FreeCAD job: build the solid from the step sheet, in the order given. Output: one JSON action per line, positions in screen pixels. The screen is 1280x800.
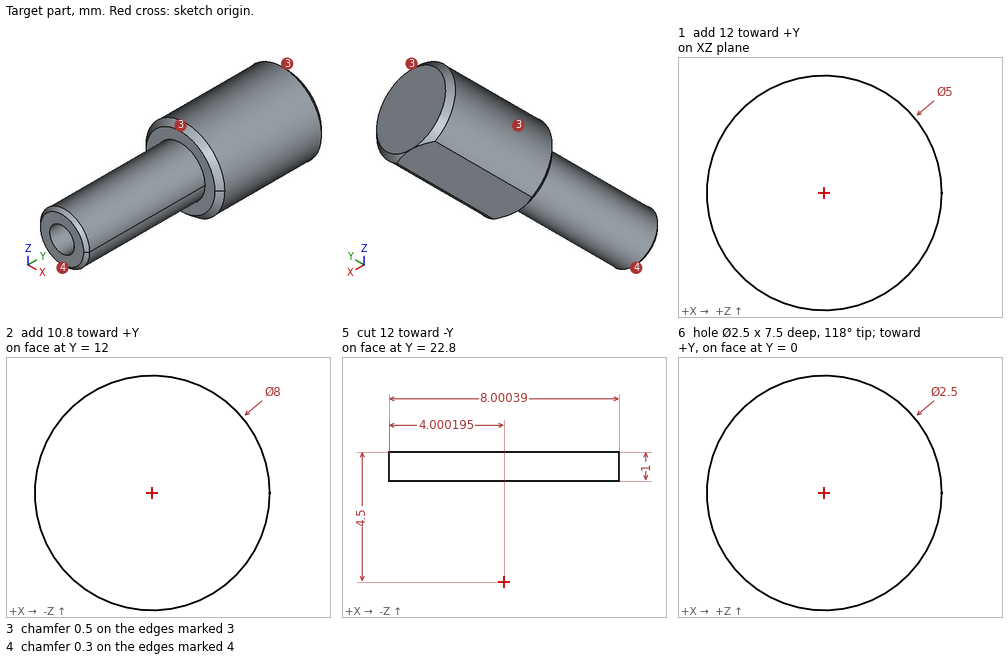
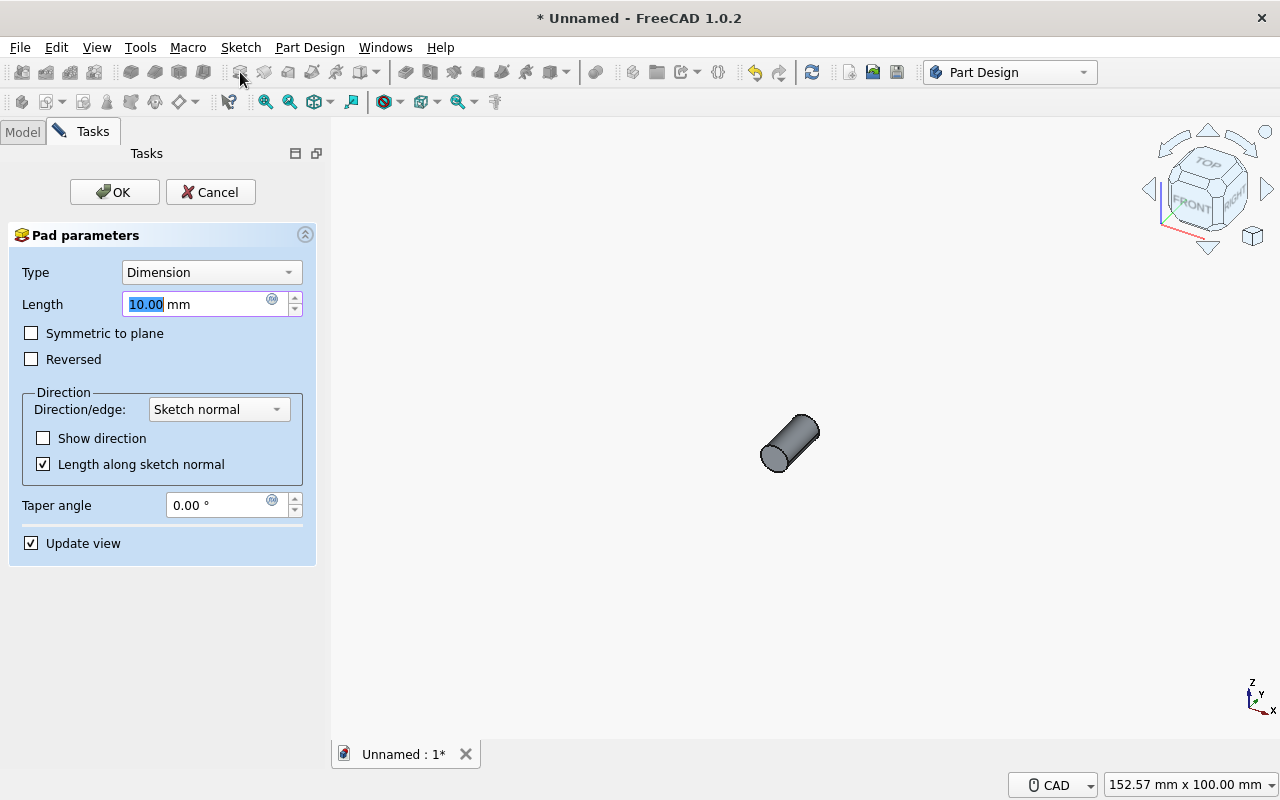
{"action": "type", "text": "12"}
{"action": "key", "text": "Tab"}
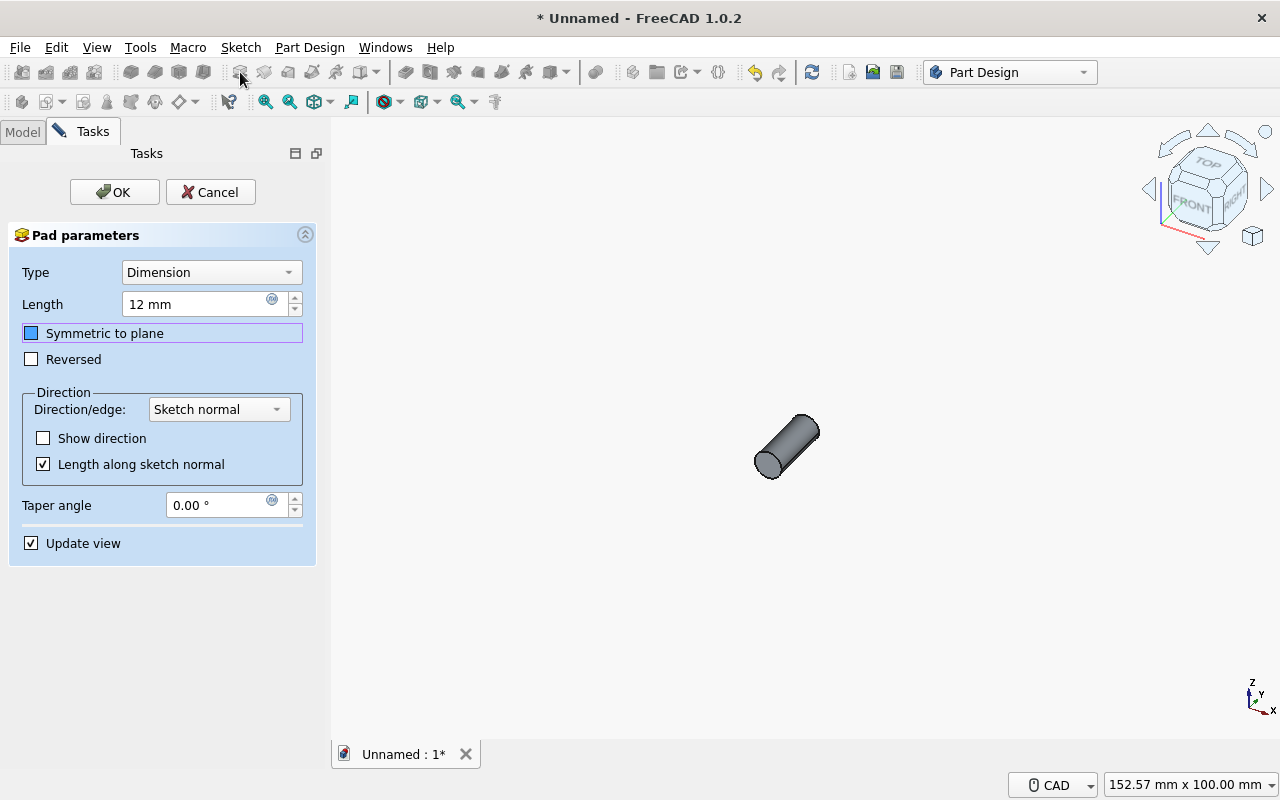
{"action": "left_click", "coordinate": [30, 359]}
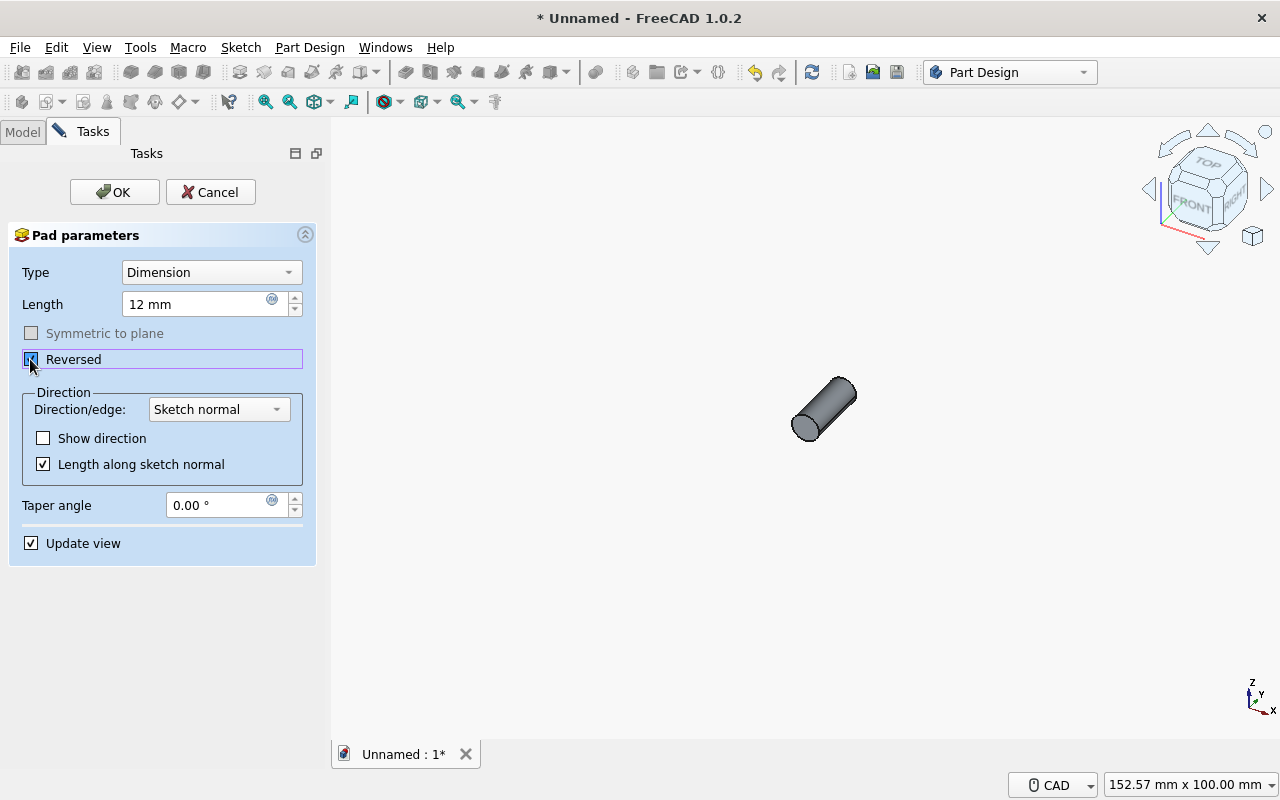
{"action": "left_click", "coordinate": [115, 192]}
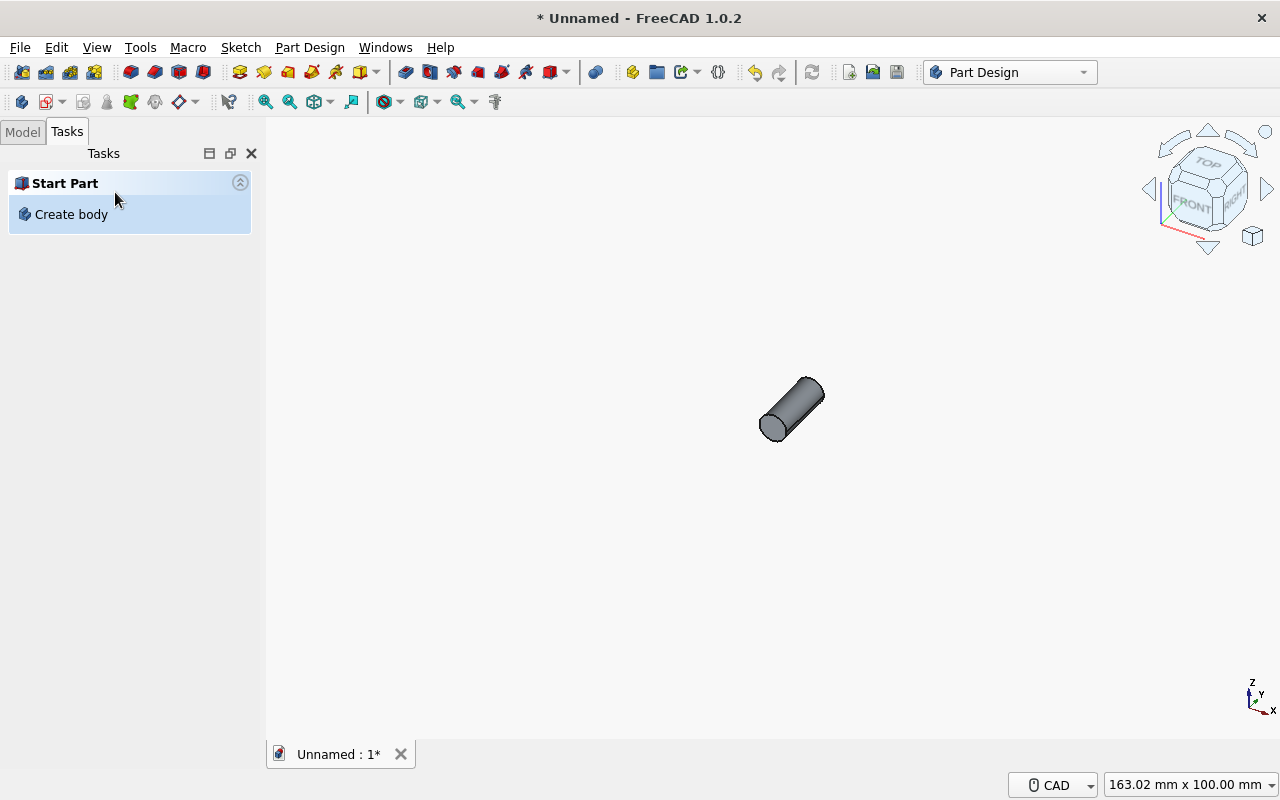
{"action": "left_click", "coordinate": [266, 102]}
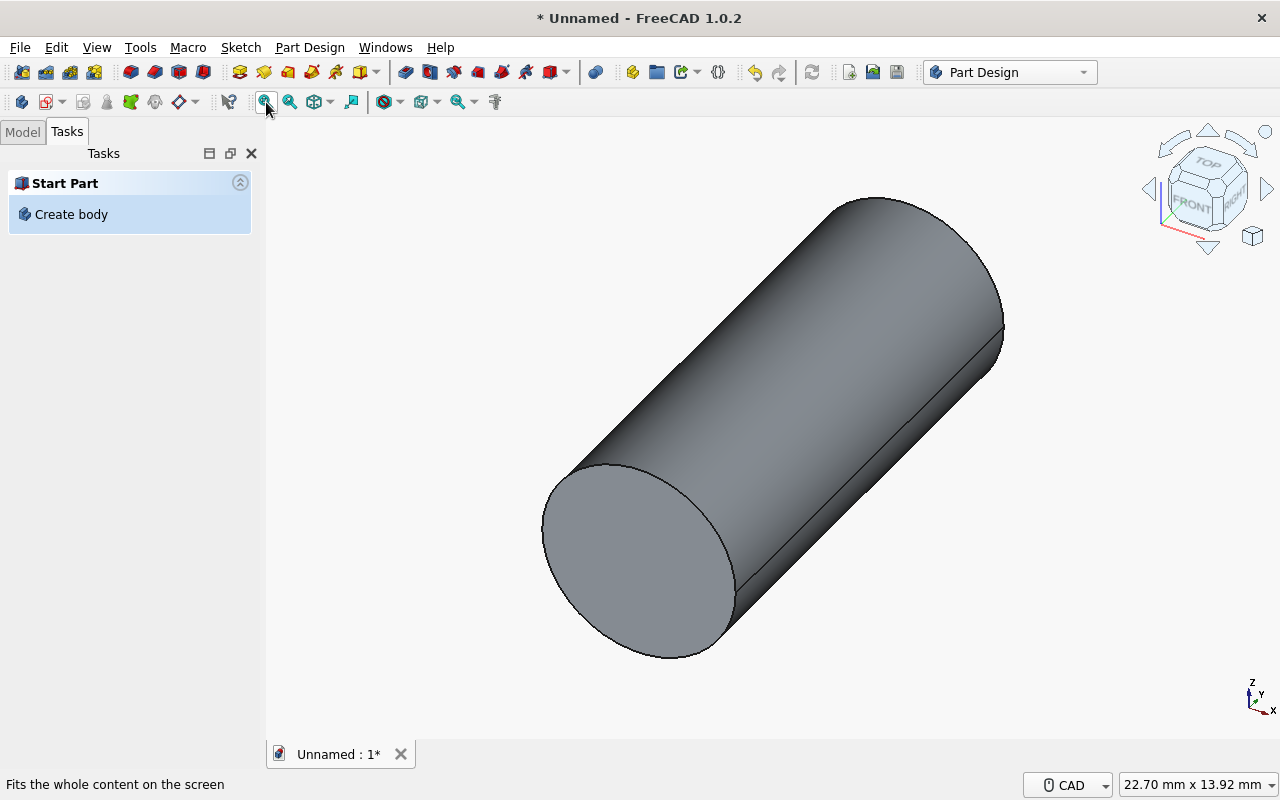
{"action": "key", "text": "4"}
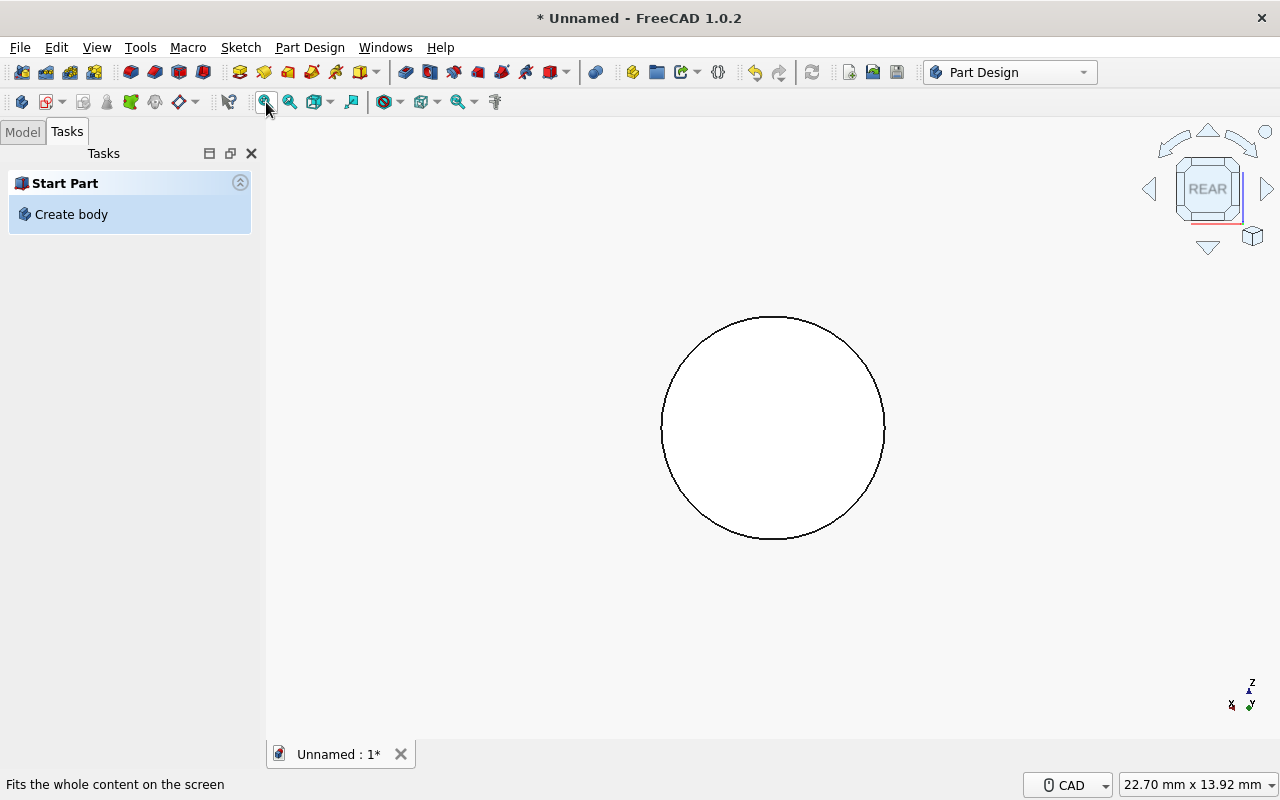
{"action": "left_click", "coordinate": [266, 102]}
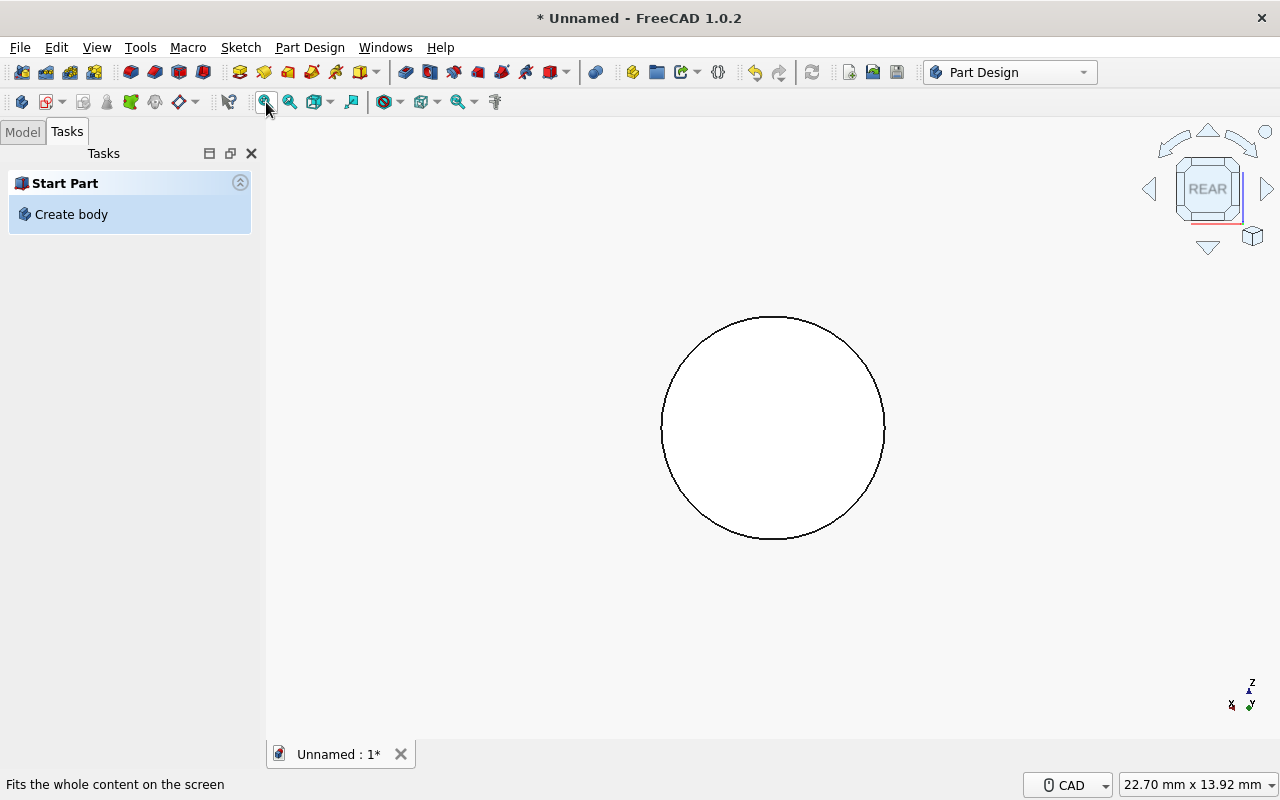
{"action": "left_click", "coordinate": [773, 427]}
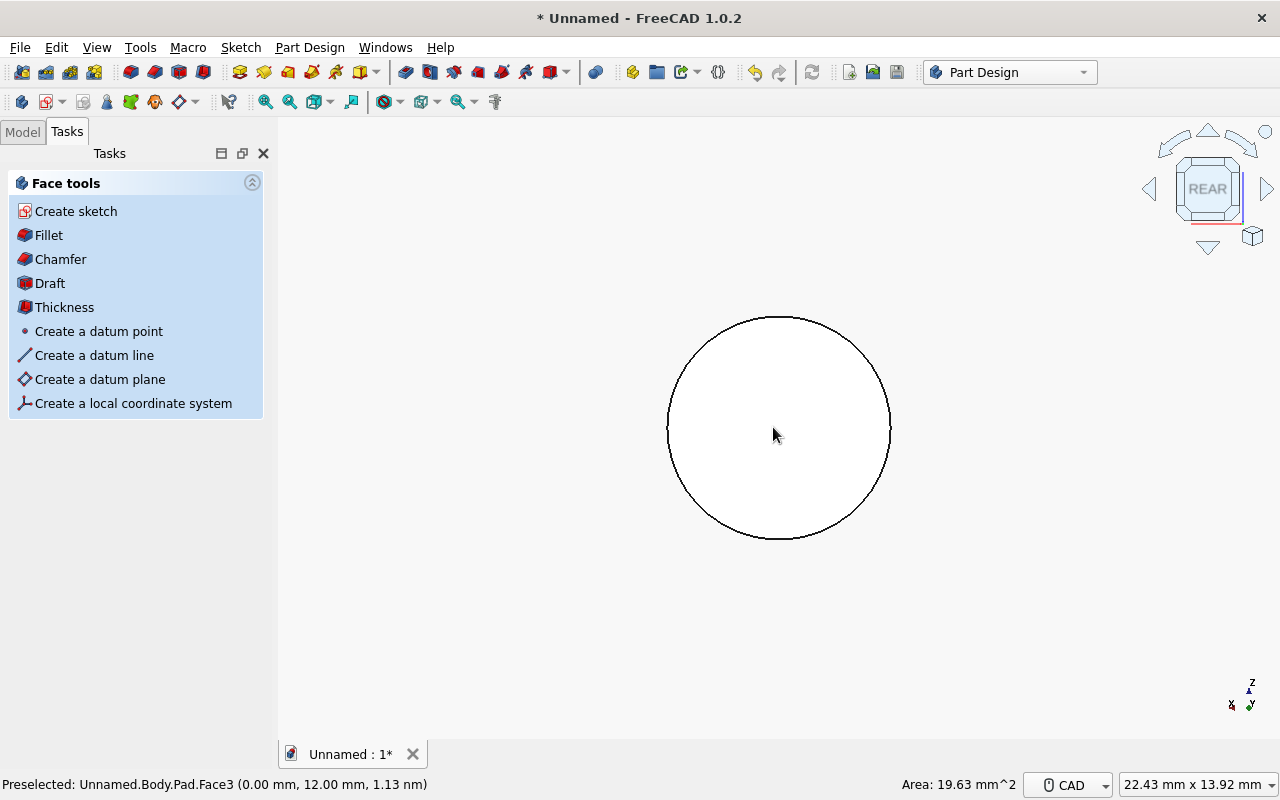
{"action": "left_click", "coordinate": [46, 102]}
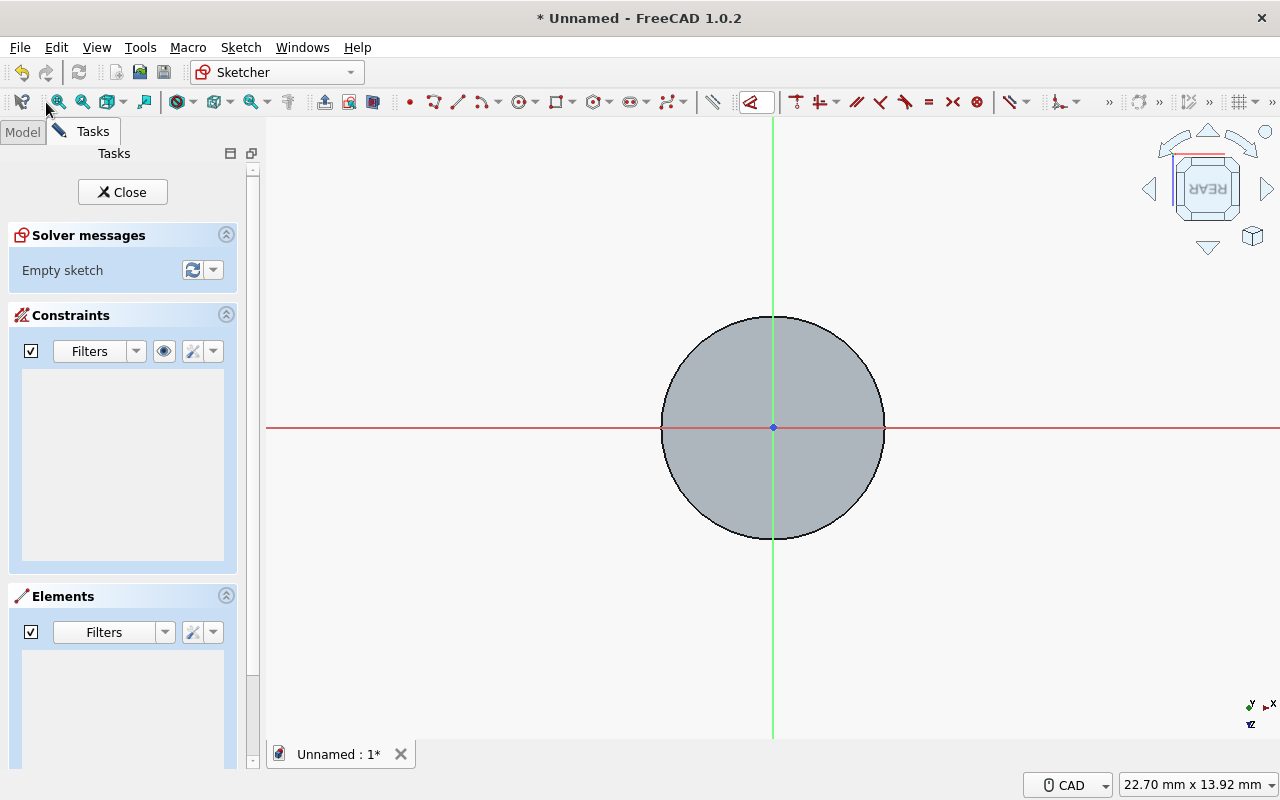
{"action": "left_click", "coordinate": [520, 102]}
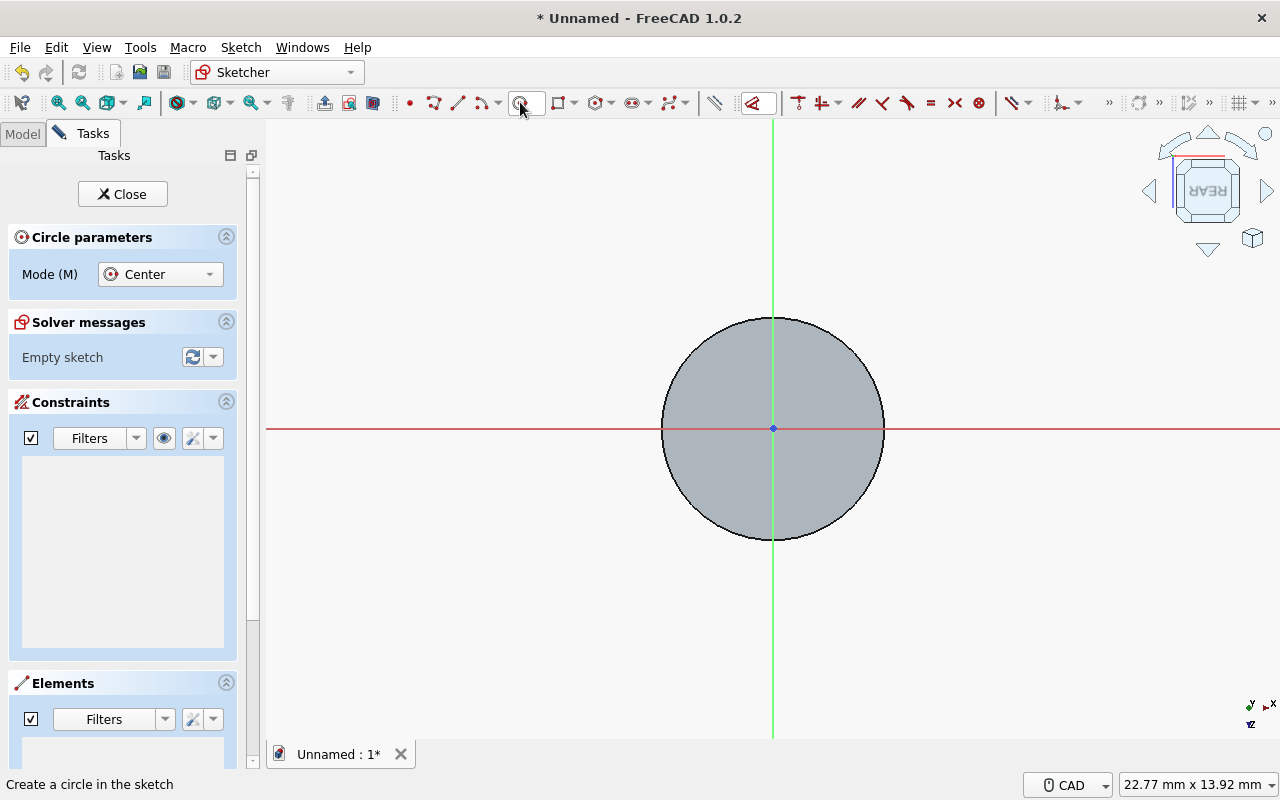
{"action": "left_click", "coordinate": [773, 429]}
{"action": "mouse_move", "coordinate": [899, 303]}